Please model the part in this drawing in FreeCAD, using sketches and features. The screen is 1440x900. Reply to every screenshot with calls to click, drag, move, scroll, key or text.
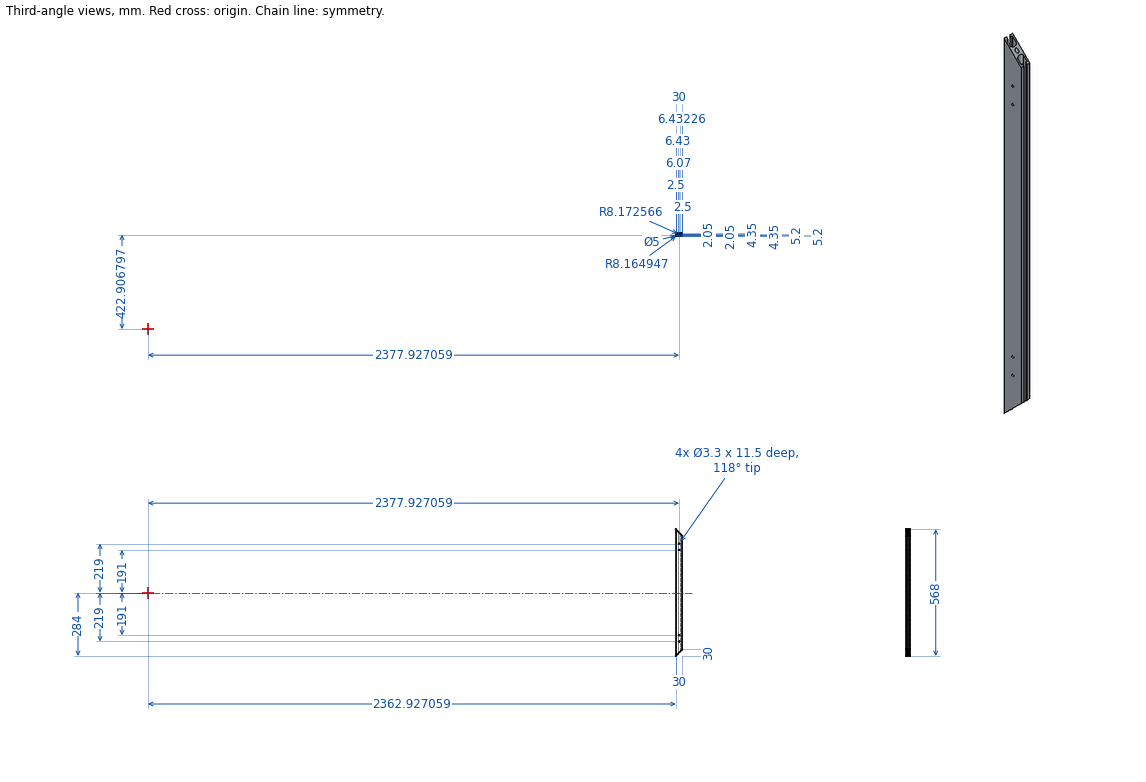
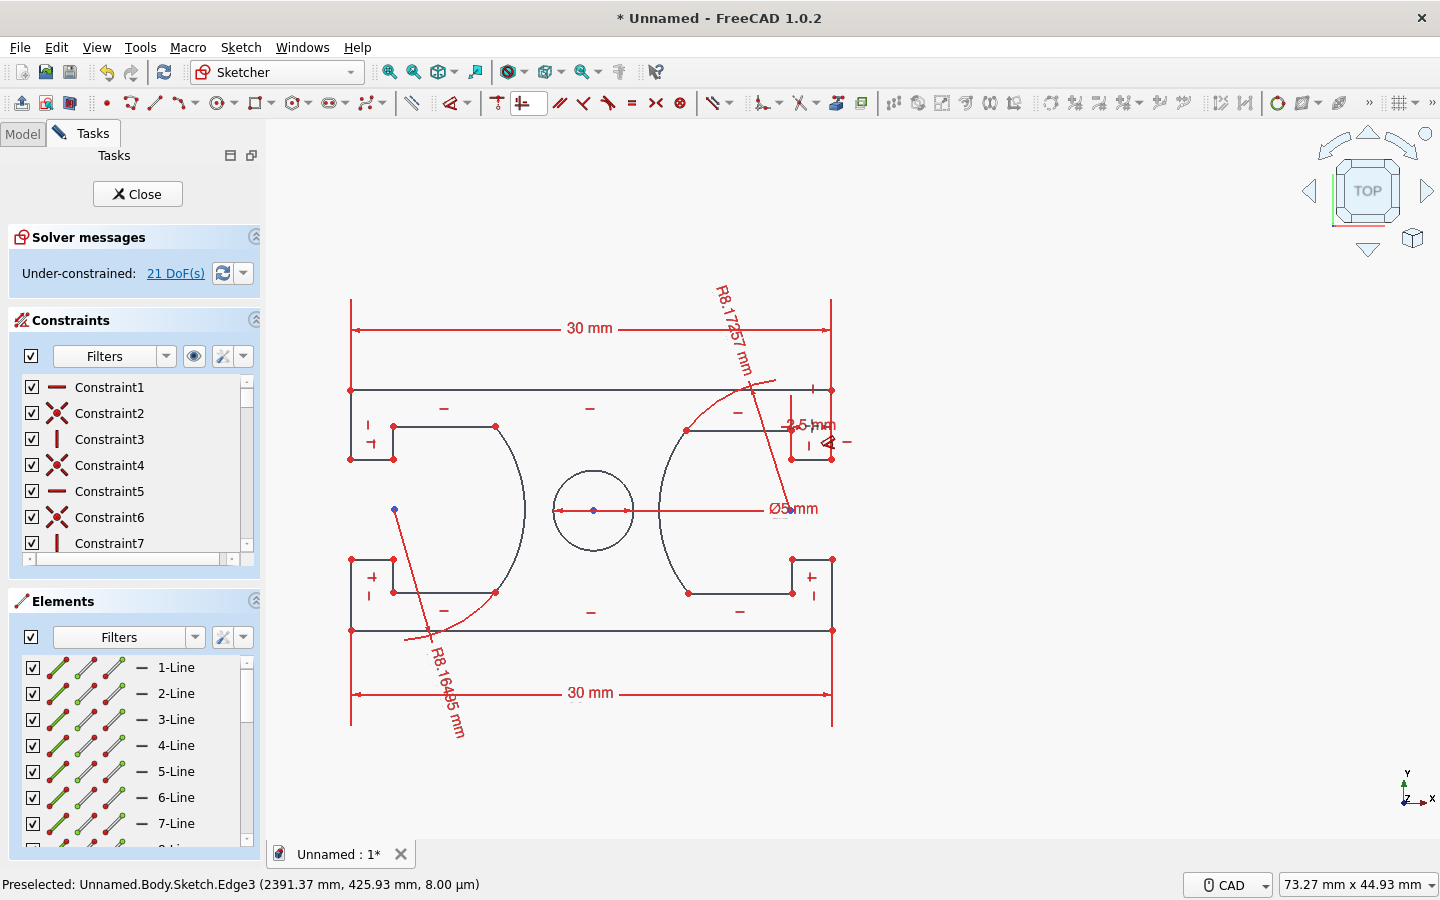
click(363, 460)
click(372, 426)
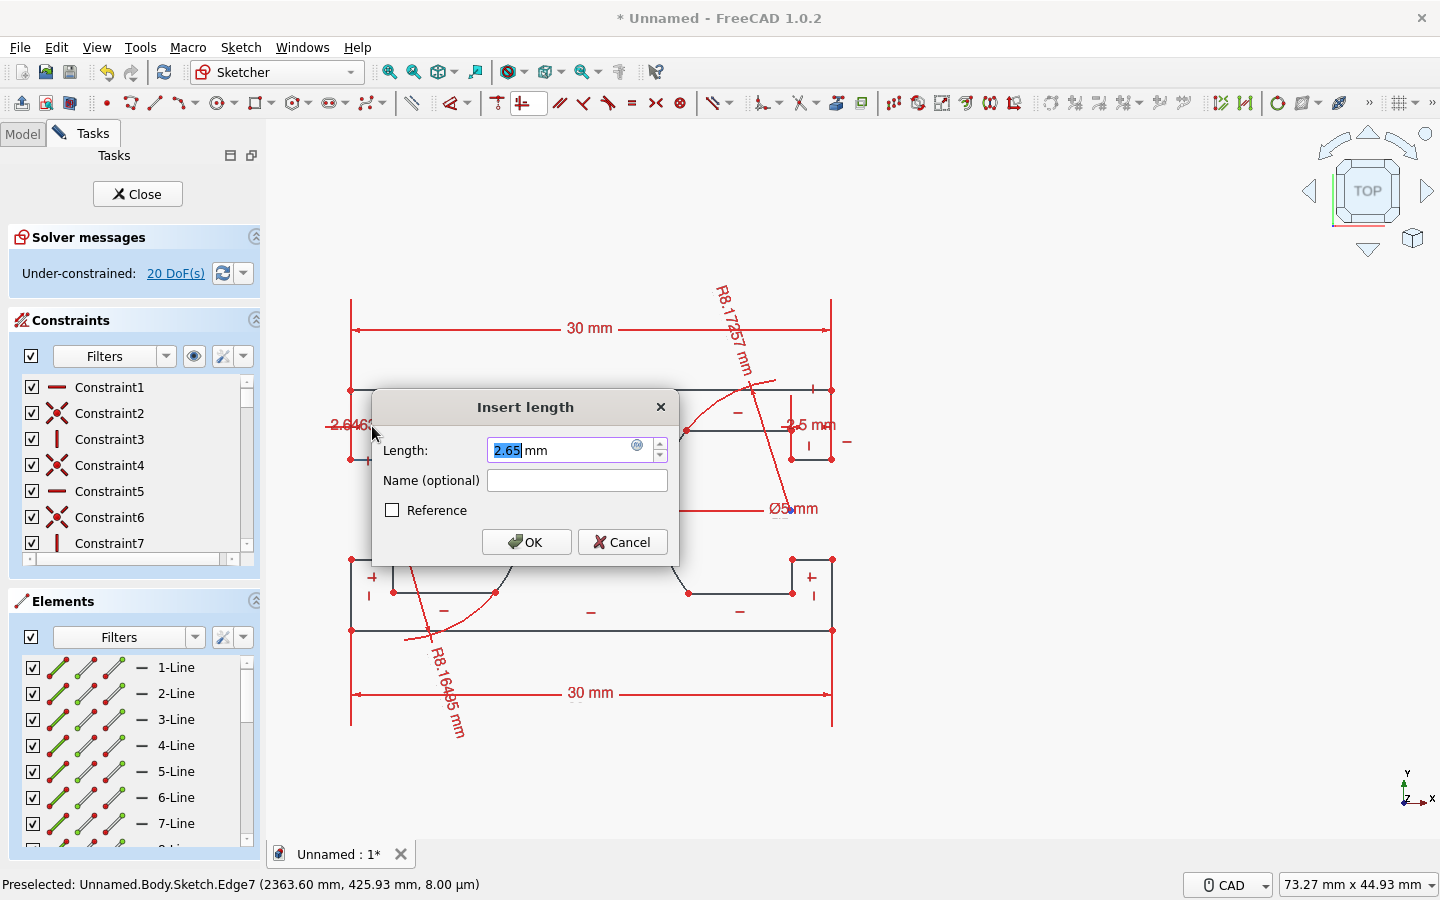
text(2.5)
key(Return)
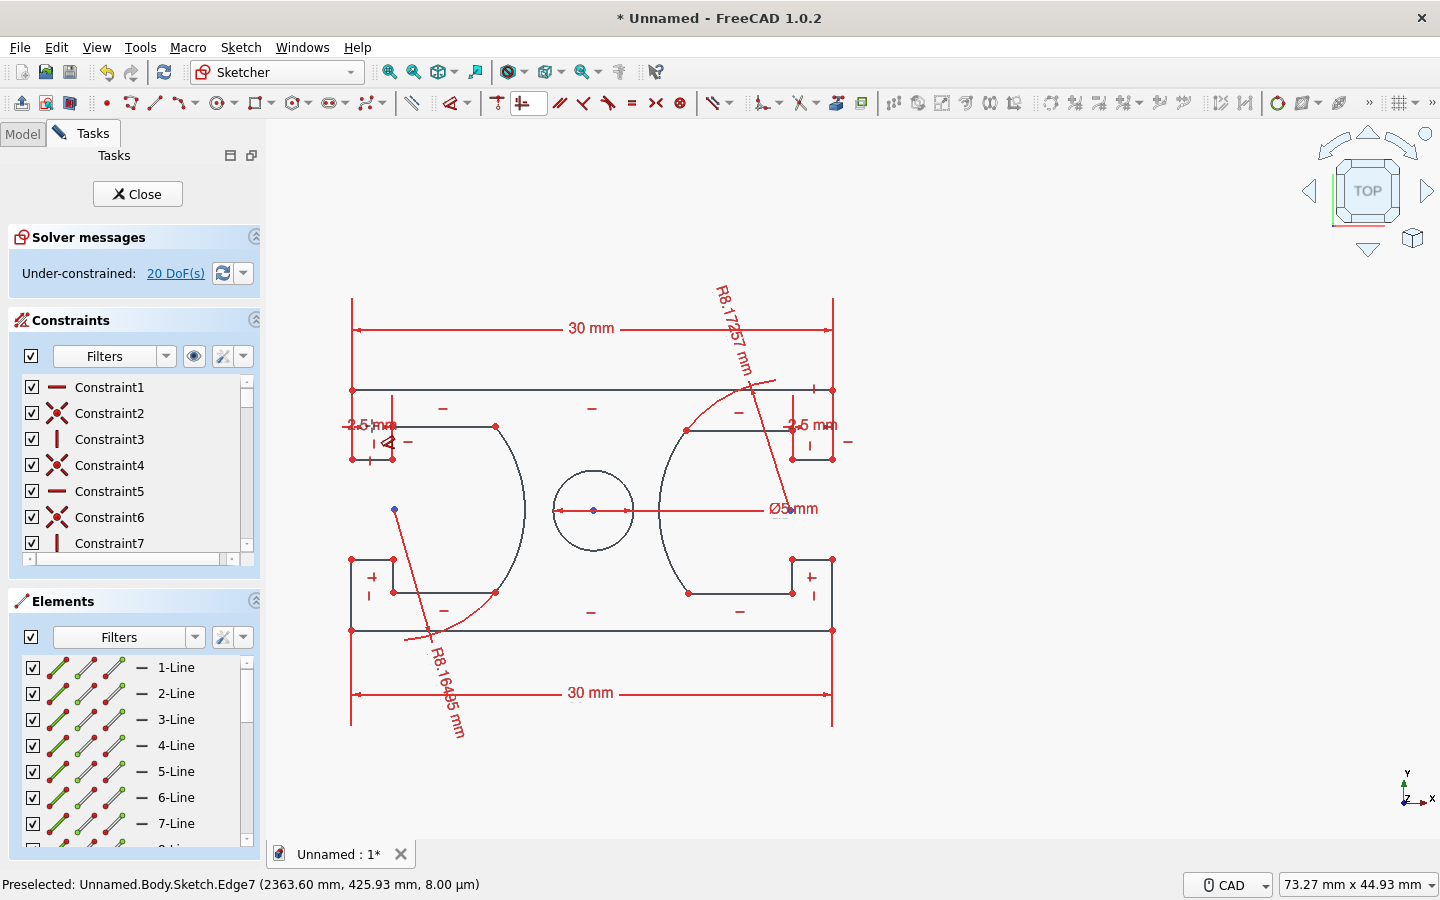
click(381, 560)
click(372, 594)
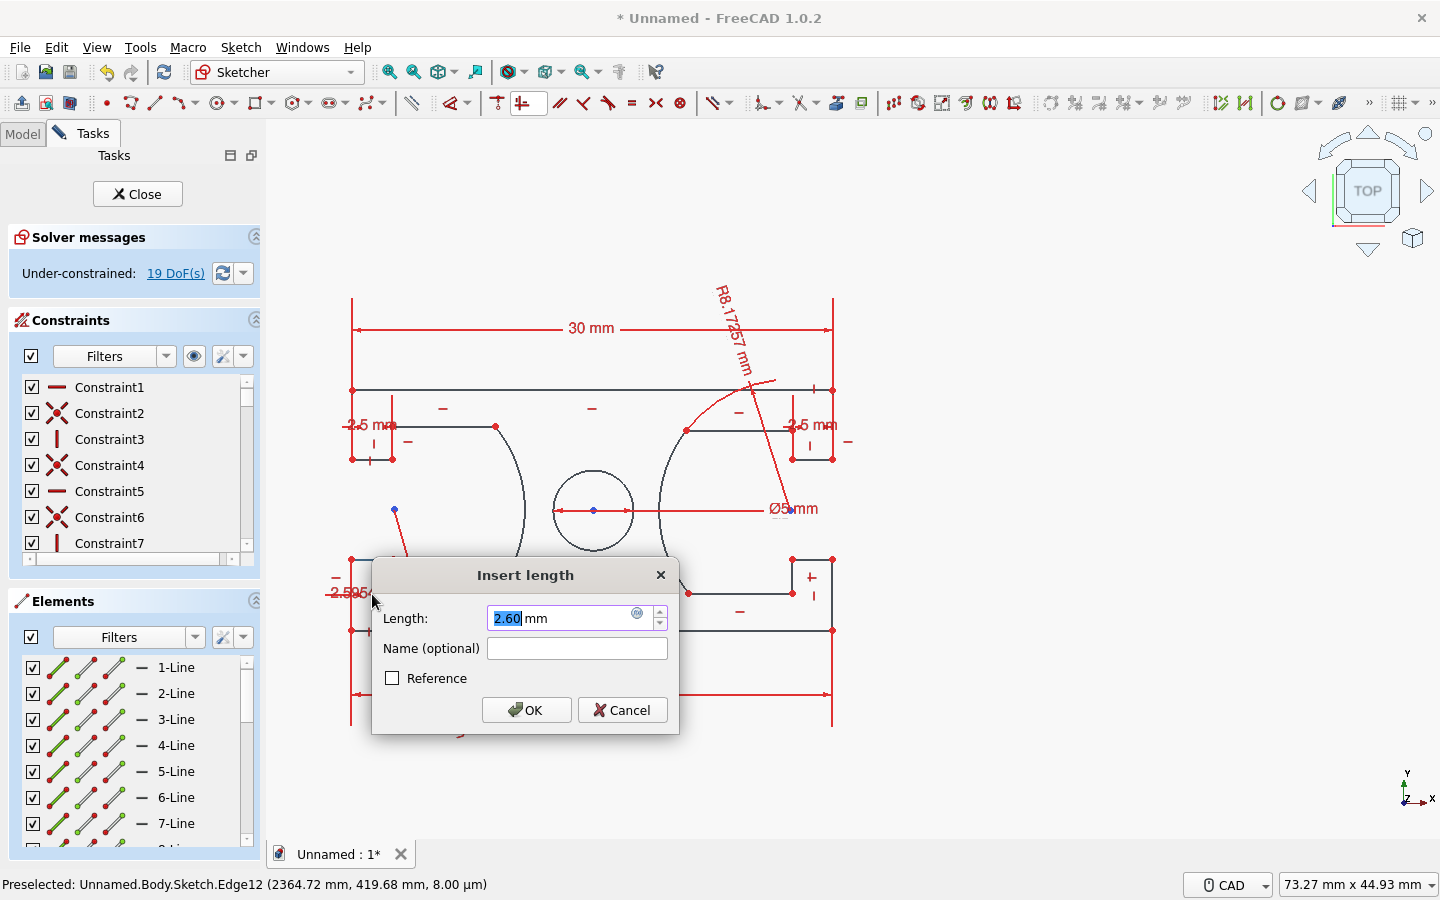
text(2.5)
key(Return)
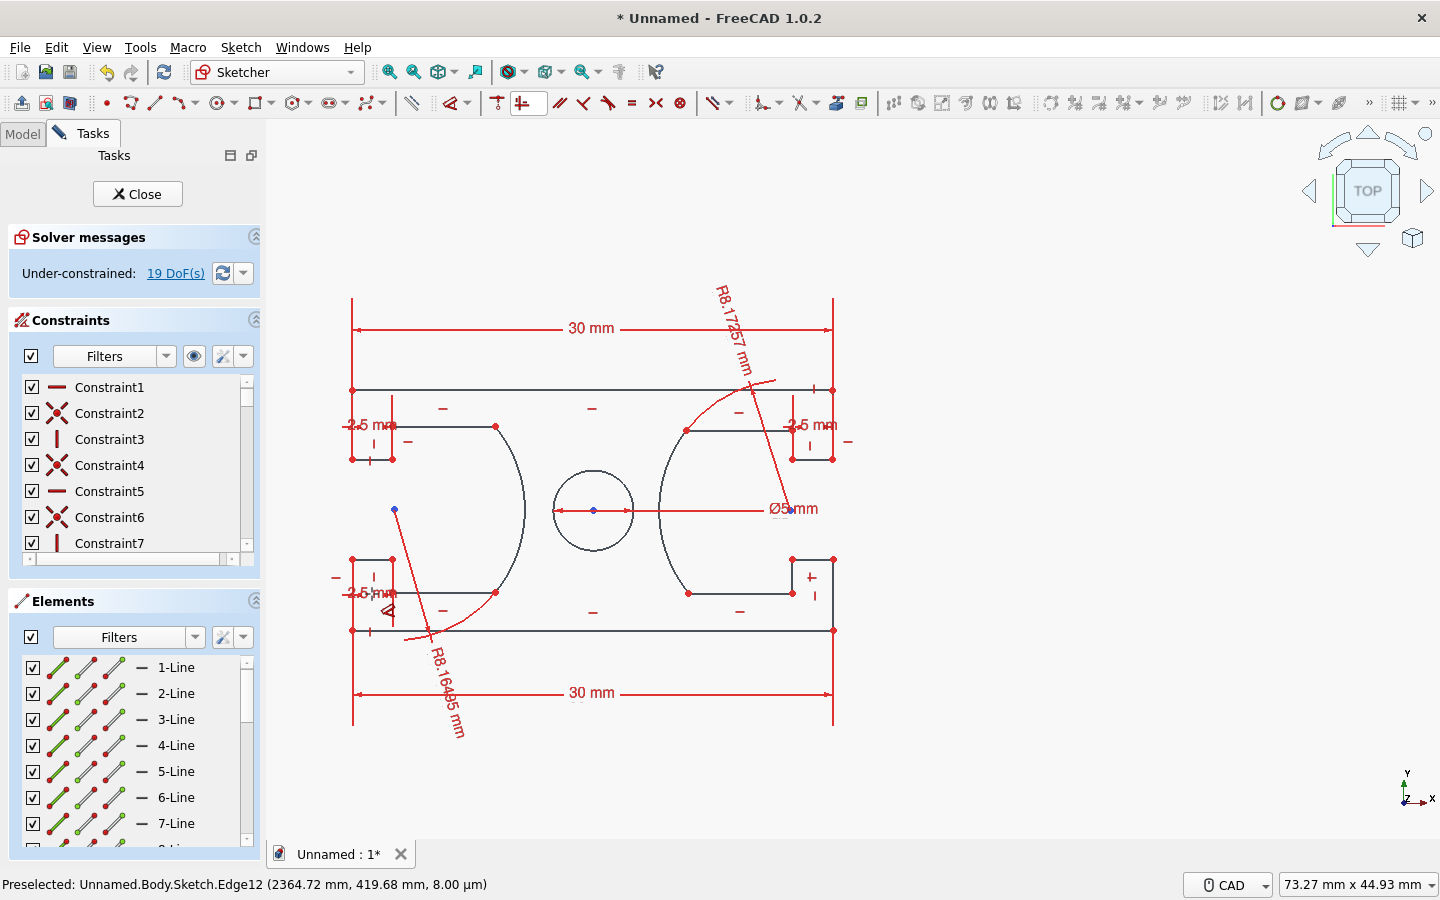
click(821, 560)
click(813, 594)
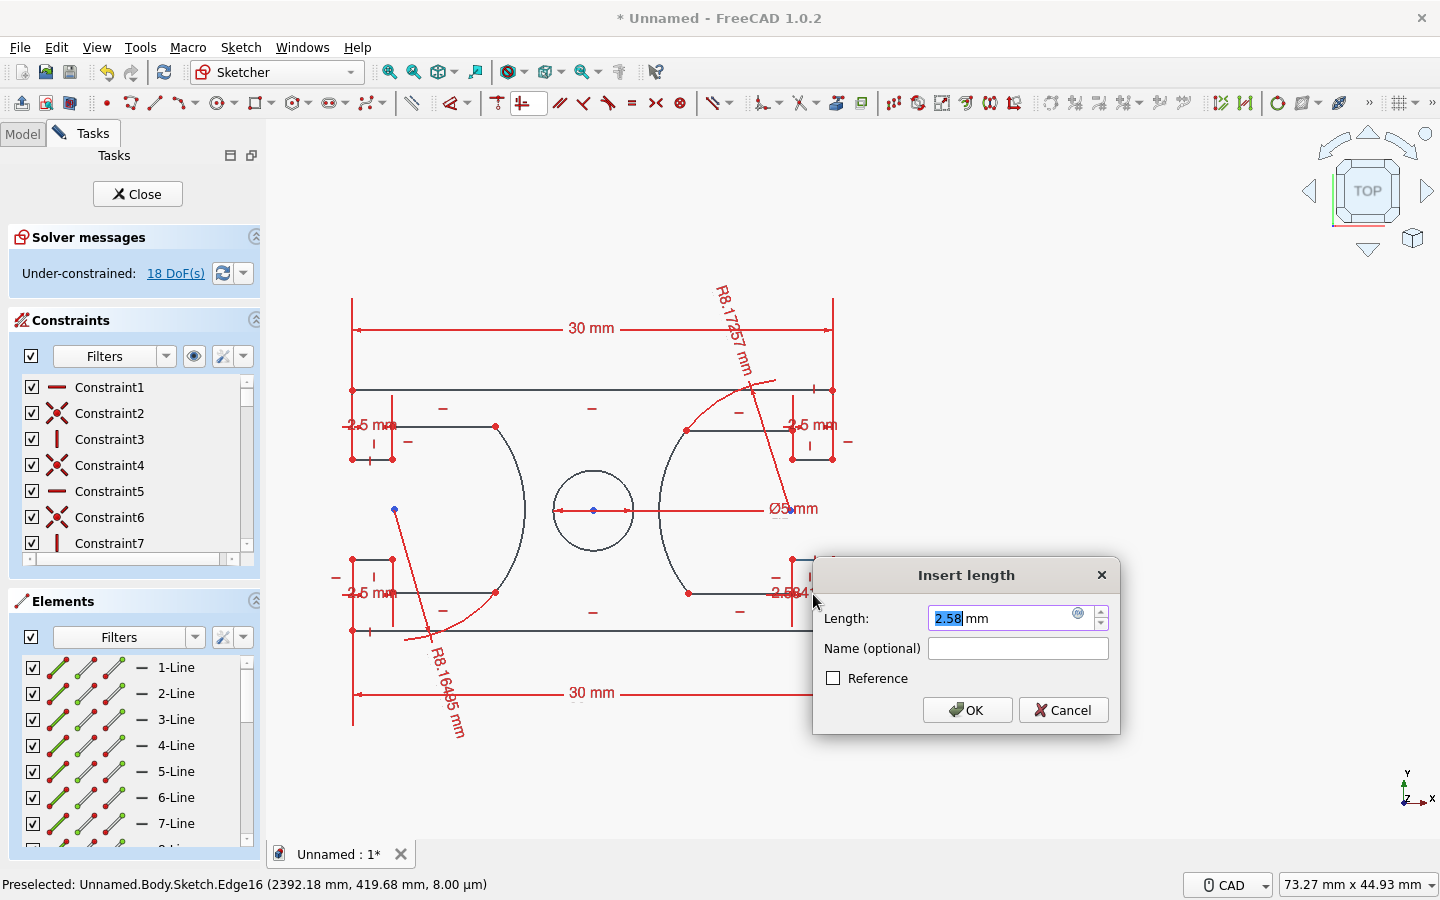
text(2.5)
key(Return)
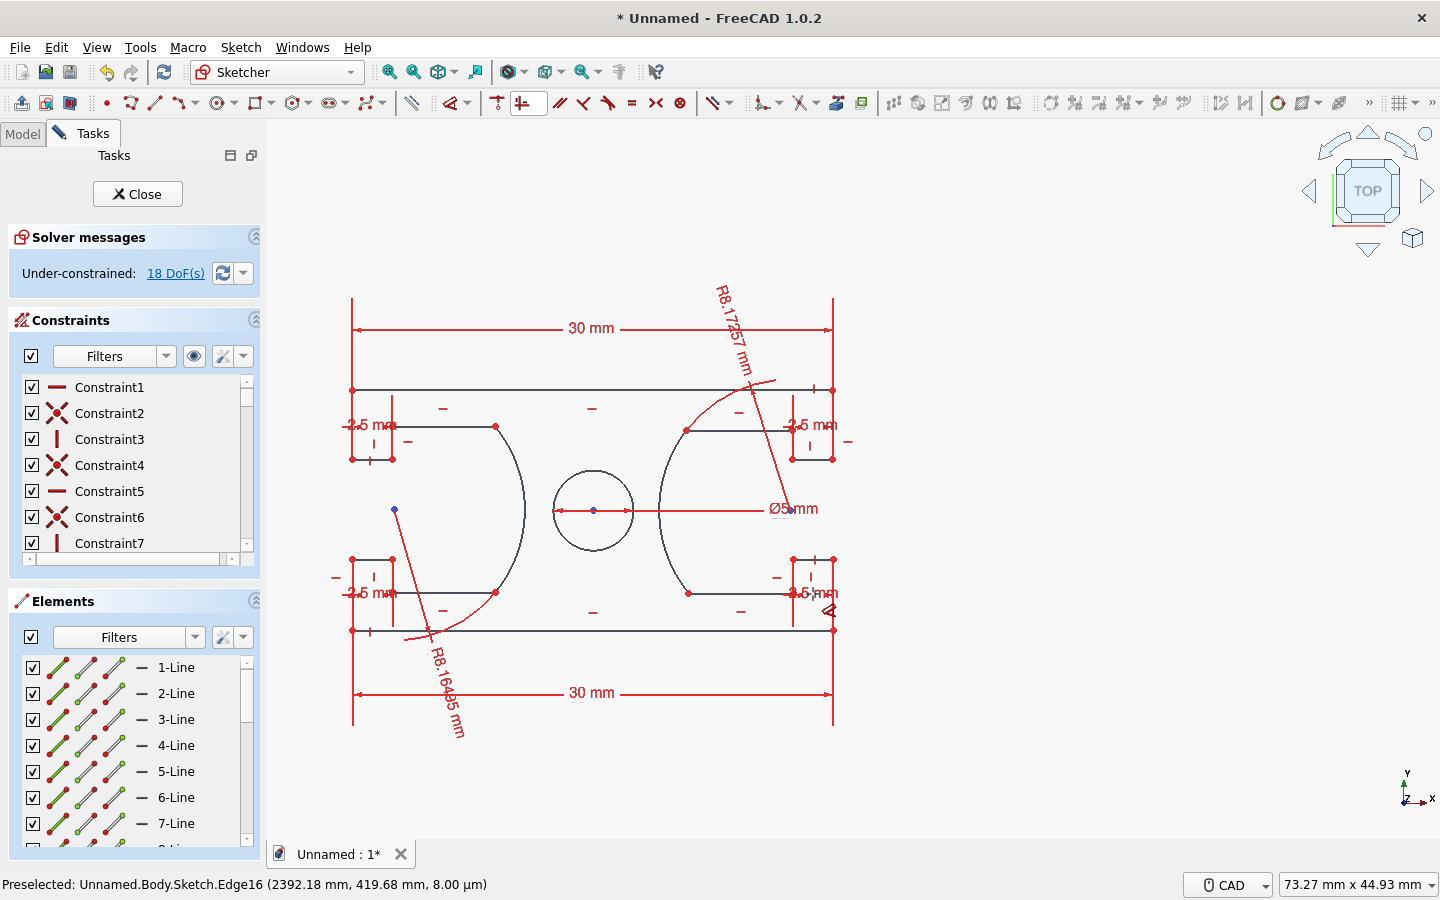
click(793, 442)
click(759, 452)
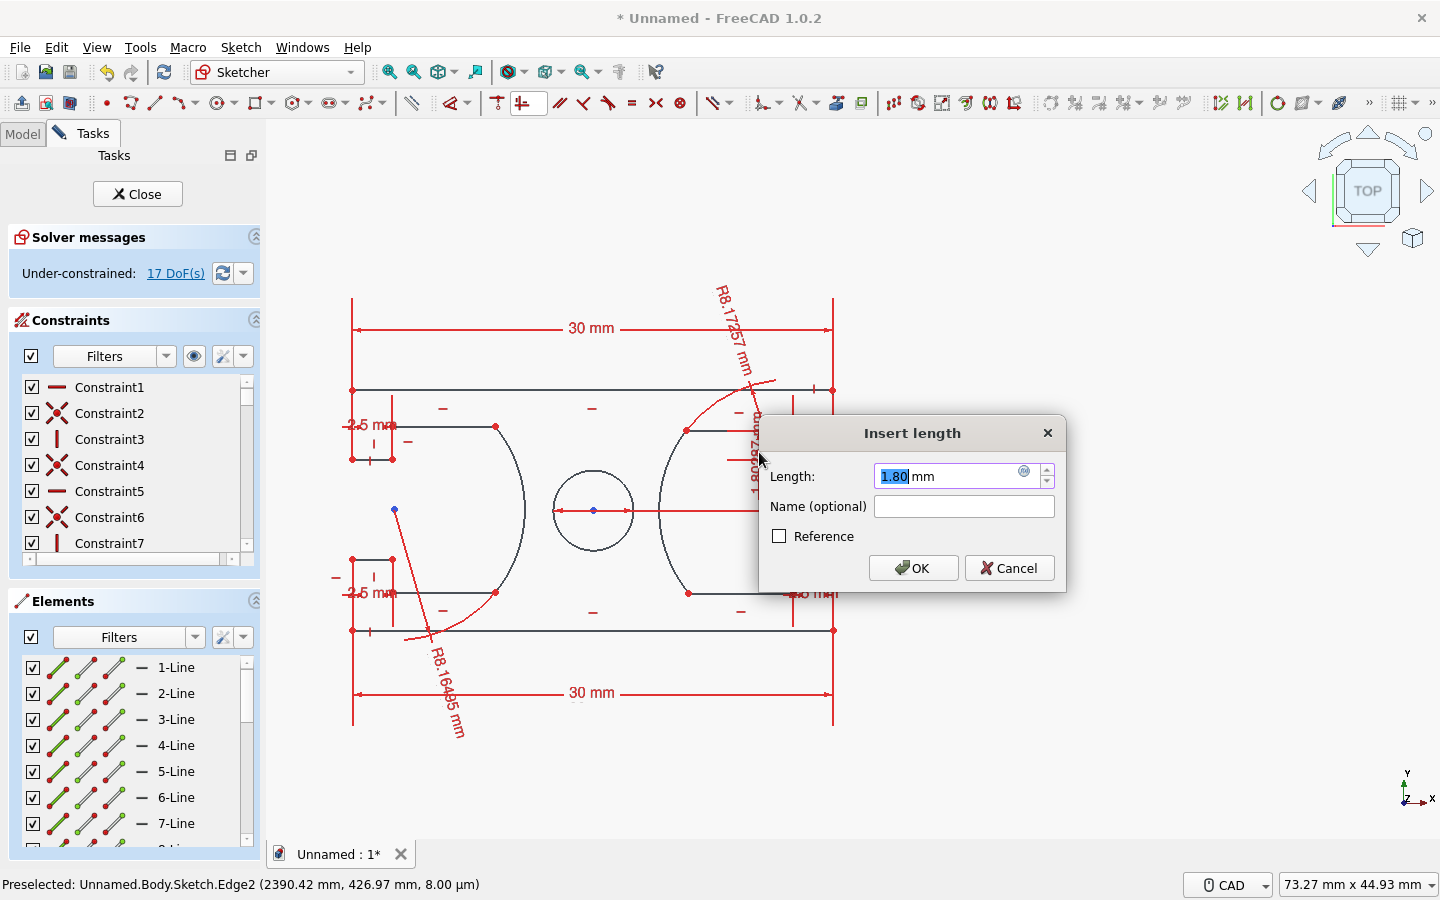
text(2.05)
key(Return)